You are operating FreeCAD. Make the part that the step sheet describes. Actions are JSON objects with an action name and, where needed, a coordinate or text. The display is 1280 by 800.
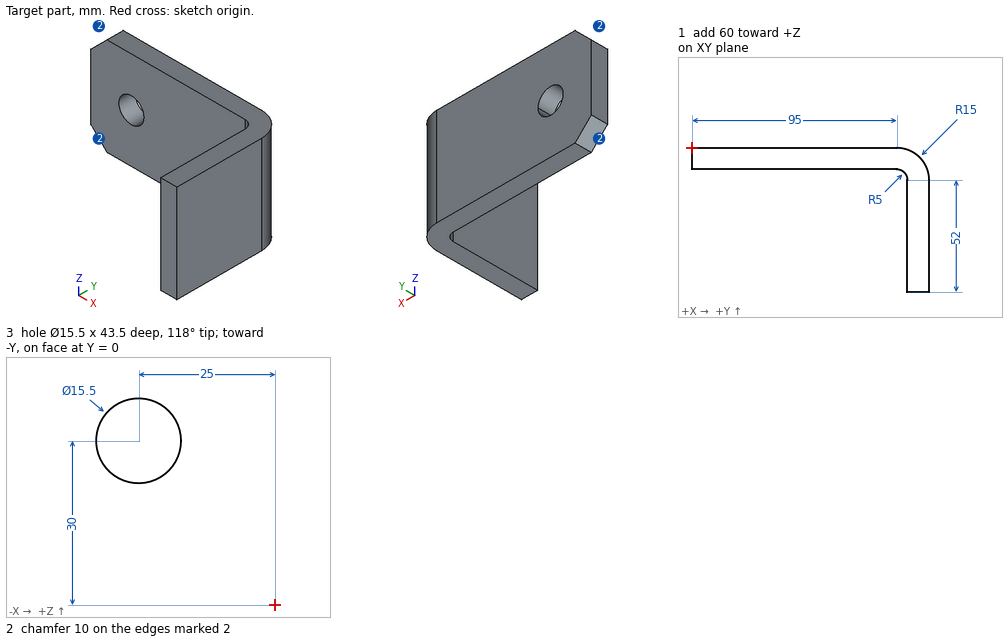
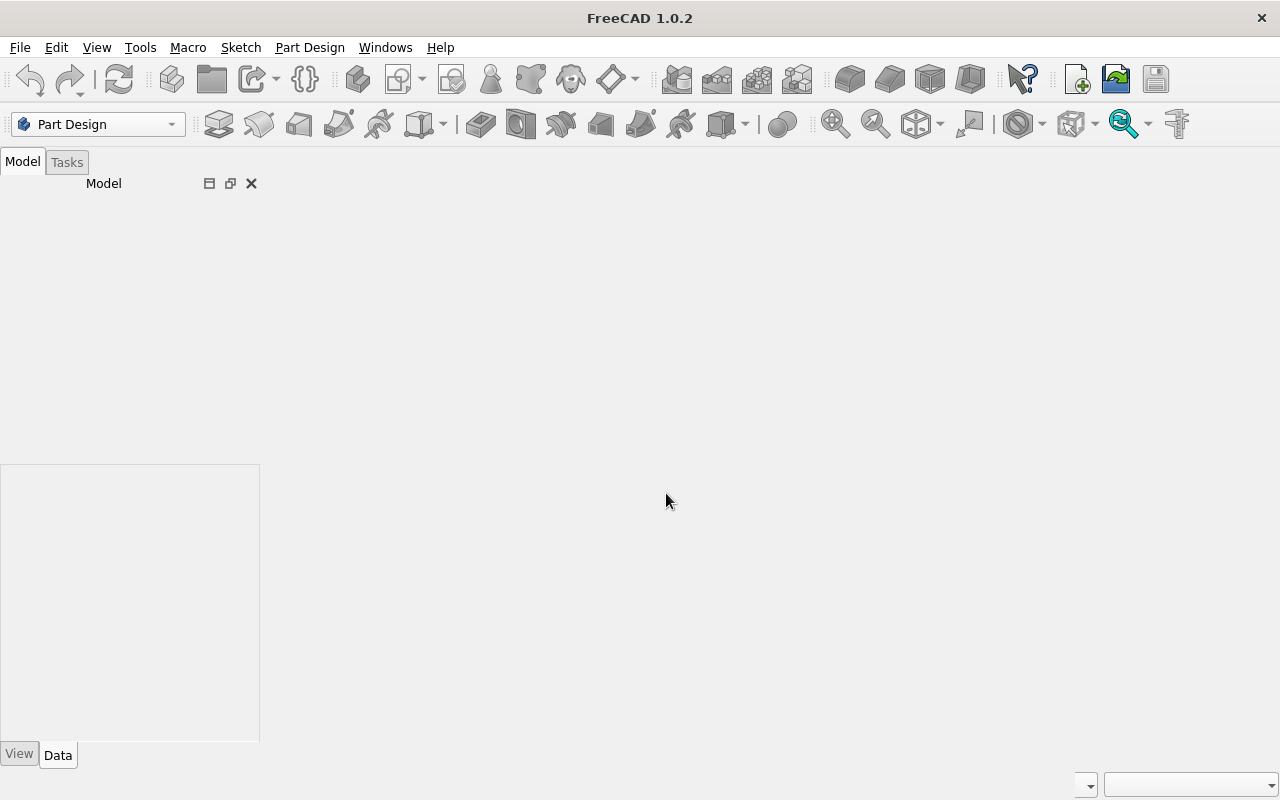
{"action": "left_click", "coordinate": [1076, 80]}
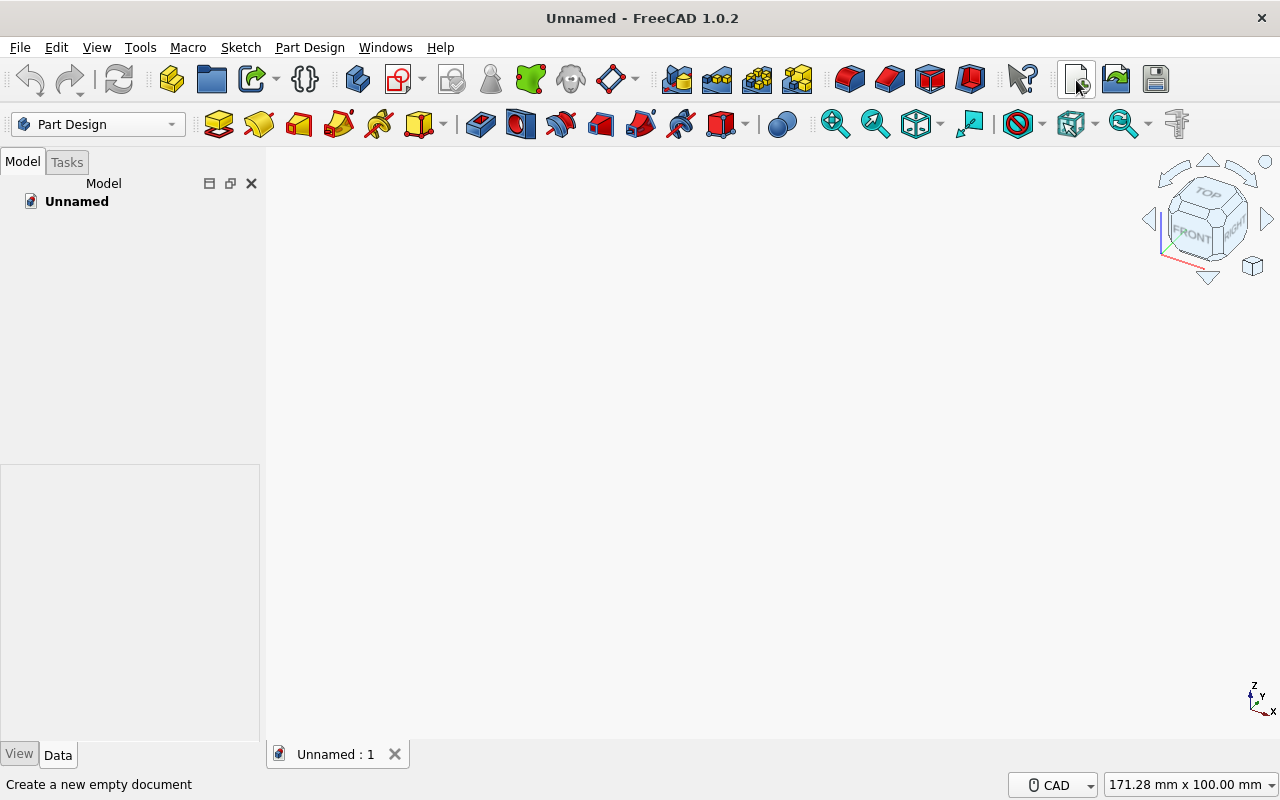
{"action": "left_click", "coordinate": [398, 80]}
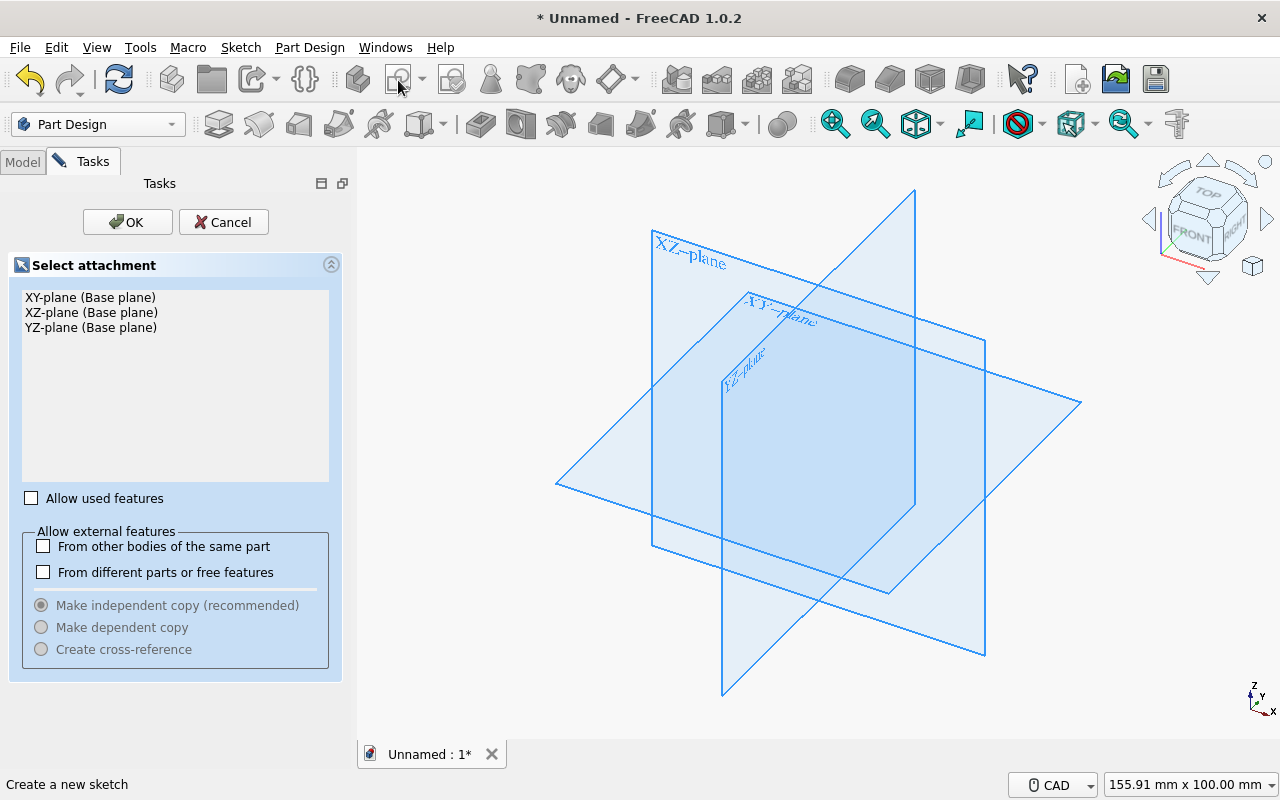
{"action": "left_click", "coordinate": [82, 298]}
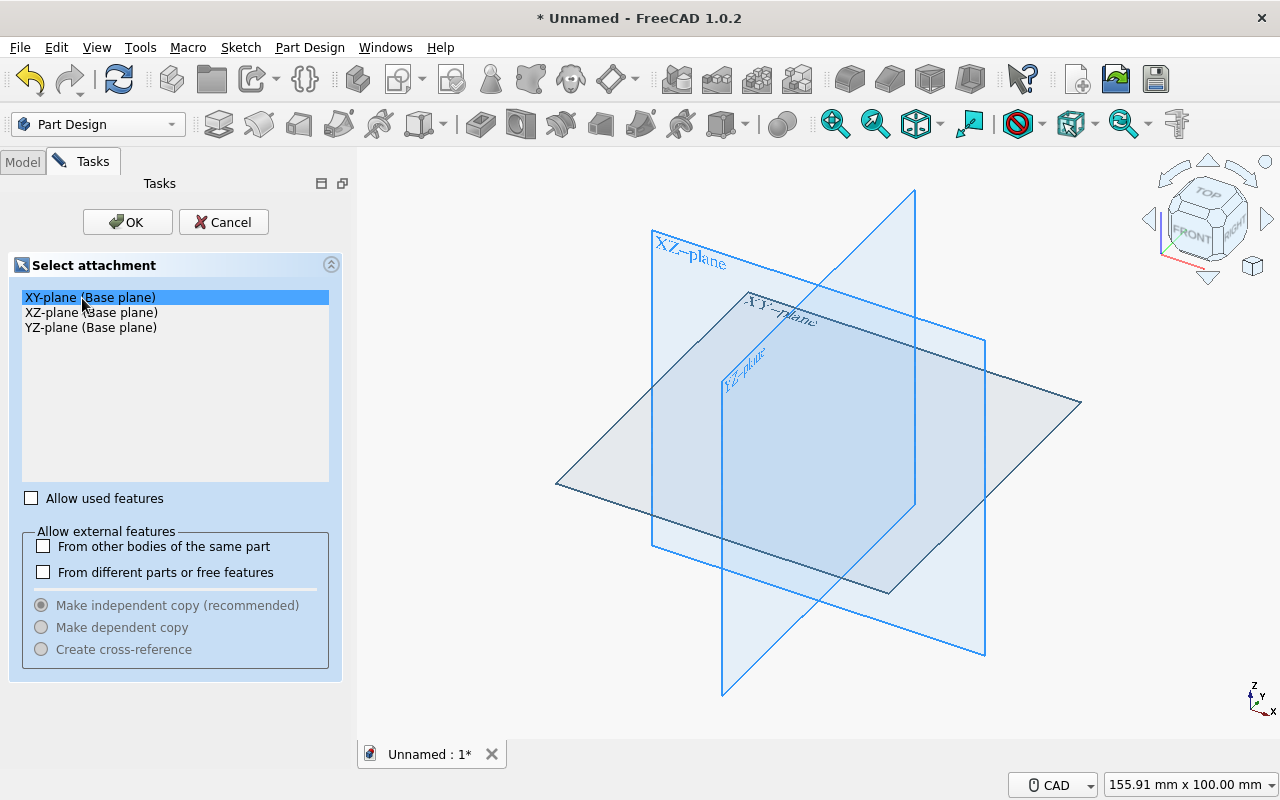
{"action": "left_click", "coordinate": [128, 222]}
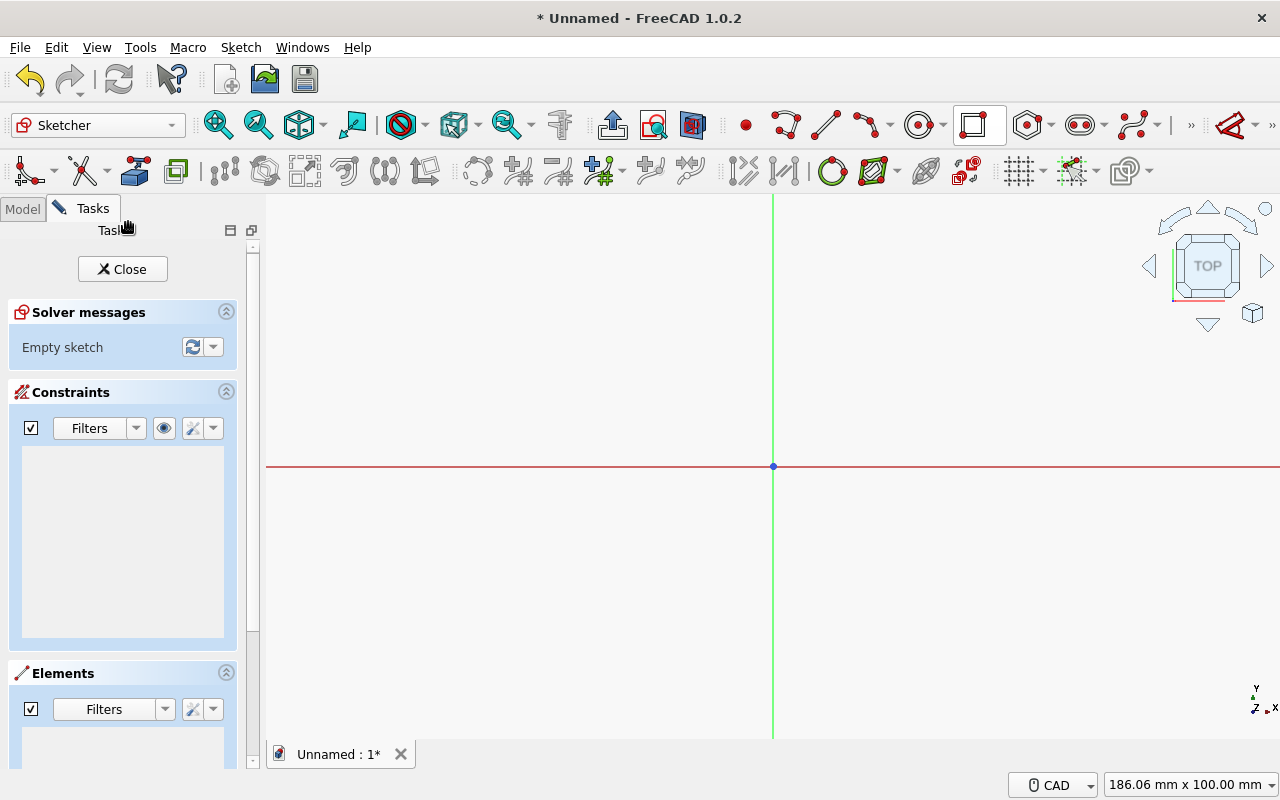
{"action": "scroll", "coordinate": [294, 222], "scroll_direction": "down", "scroll_amount": 2}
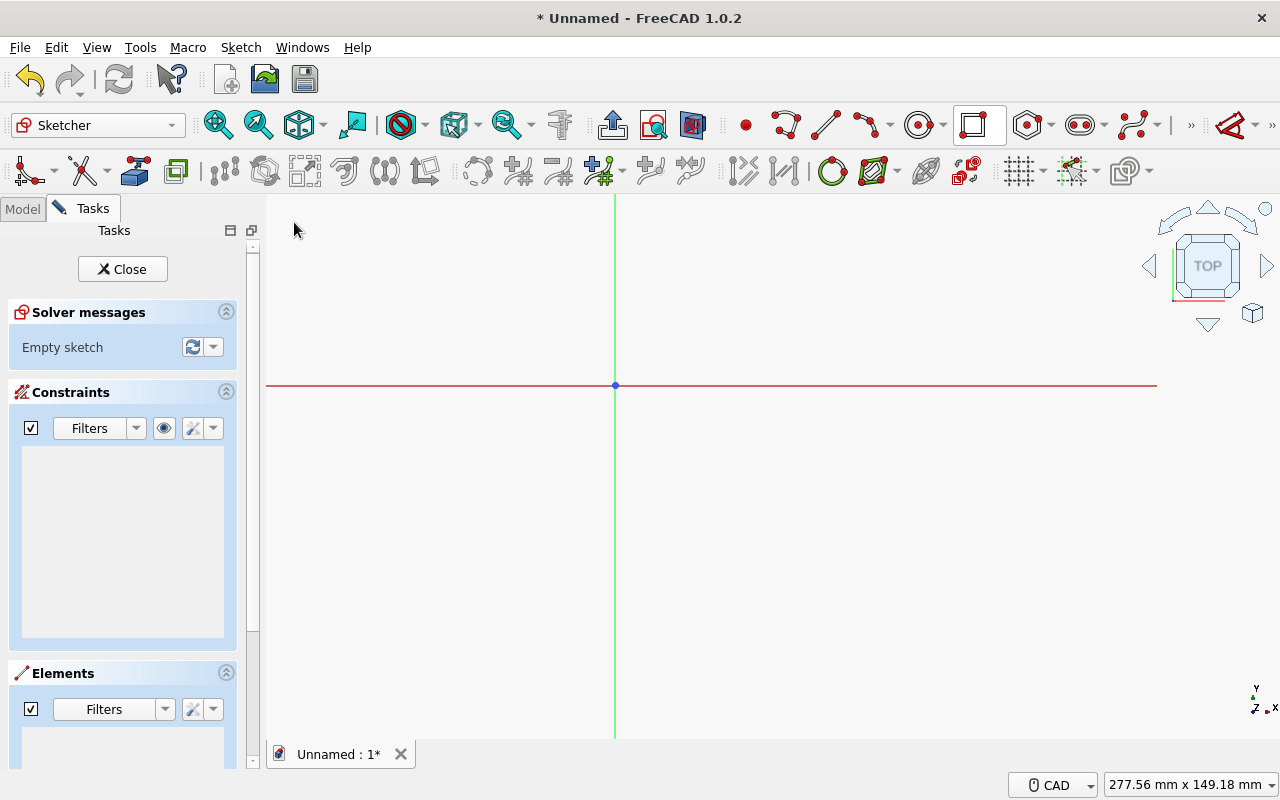
{"action": "scroll", "coordinate": [1043, 593], "scroll_direction": "up", "scroll_amount": 2}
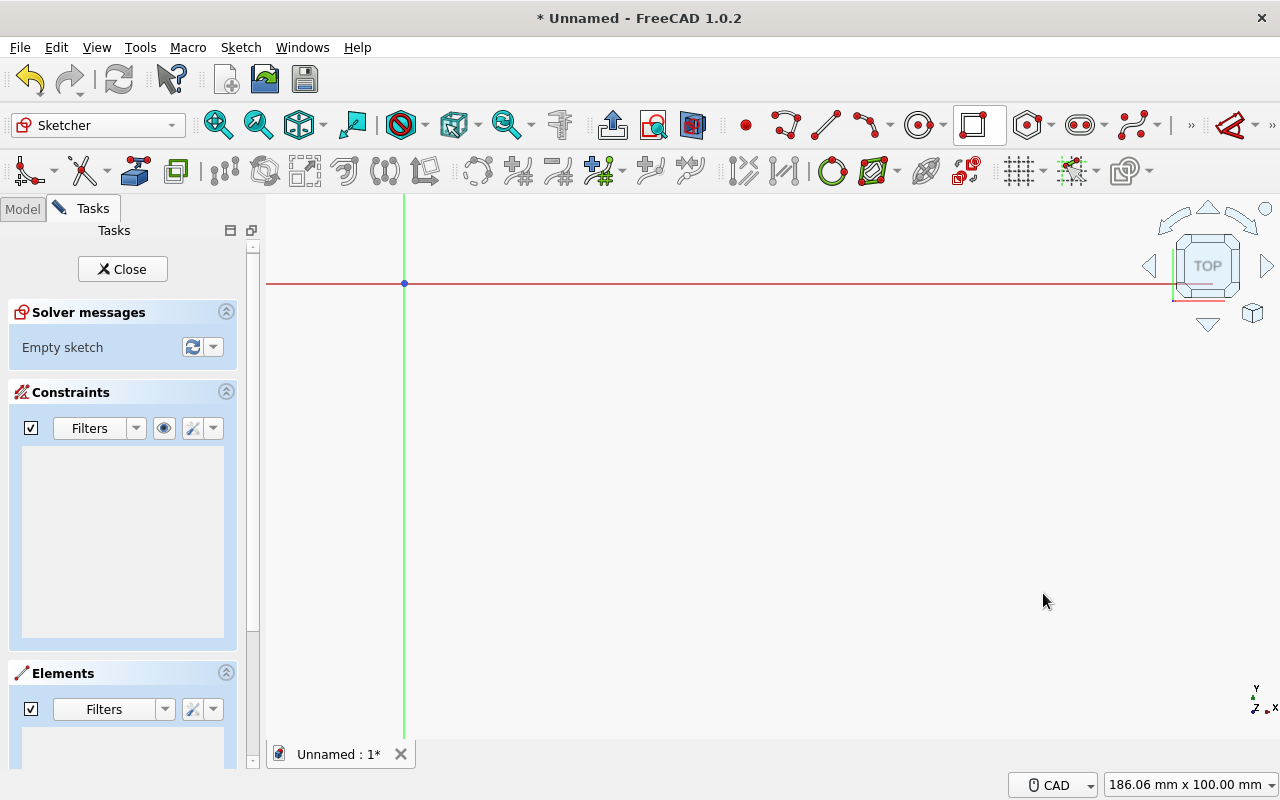
{"action": "left_click", "coordinate": [786, 126]}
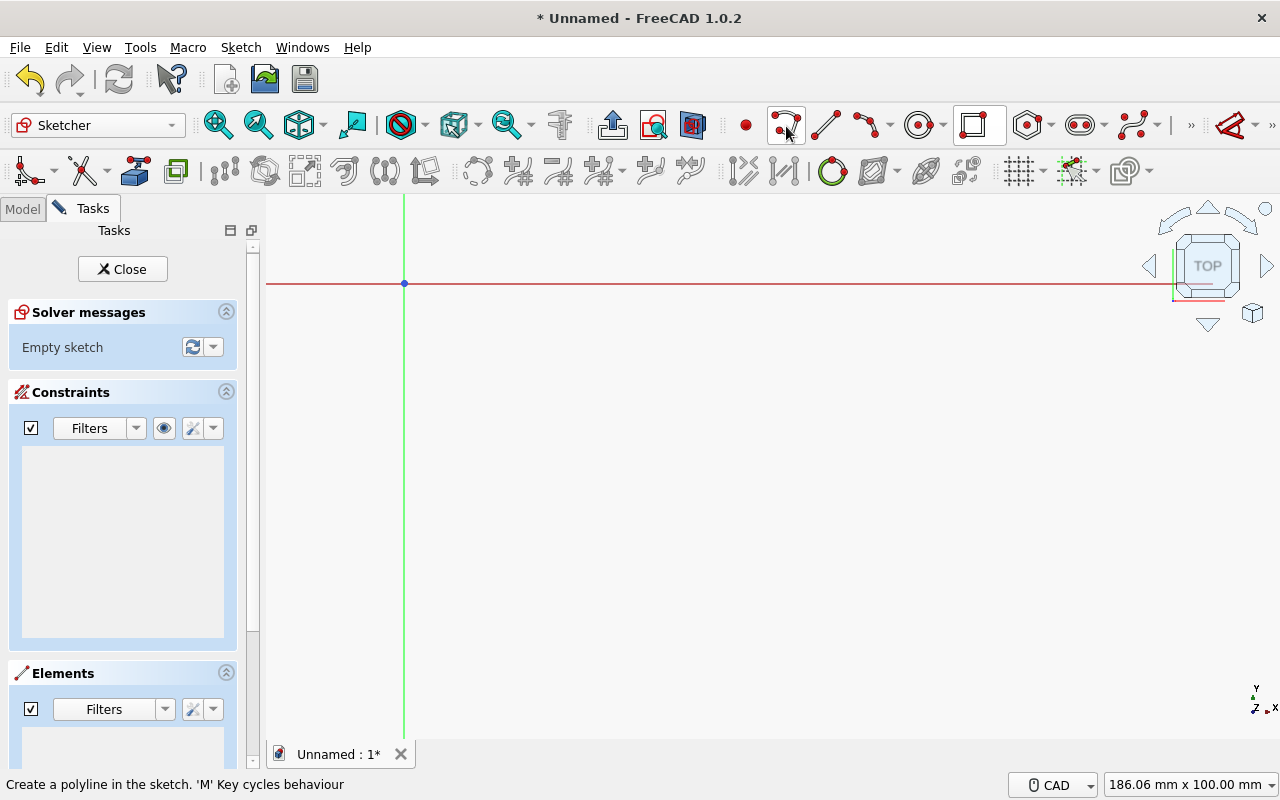
{"action": "left_click", "coordinate": [922, 284]}
{"action": "left_click", "coordinate": [404, 284]}
{"action": "left_click", "coordinate": [413, 338]}
{"action": "left_click", "coordinate": [922, 338]}
{"action": "right_click", "coordinate": [922, 338]}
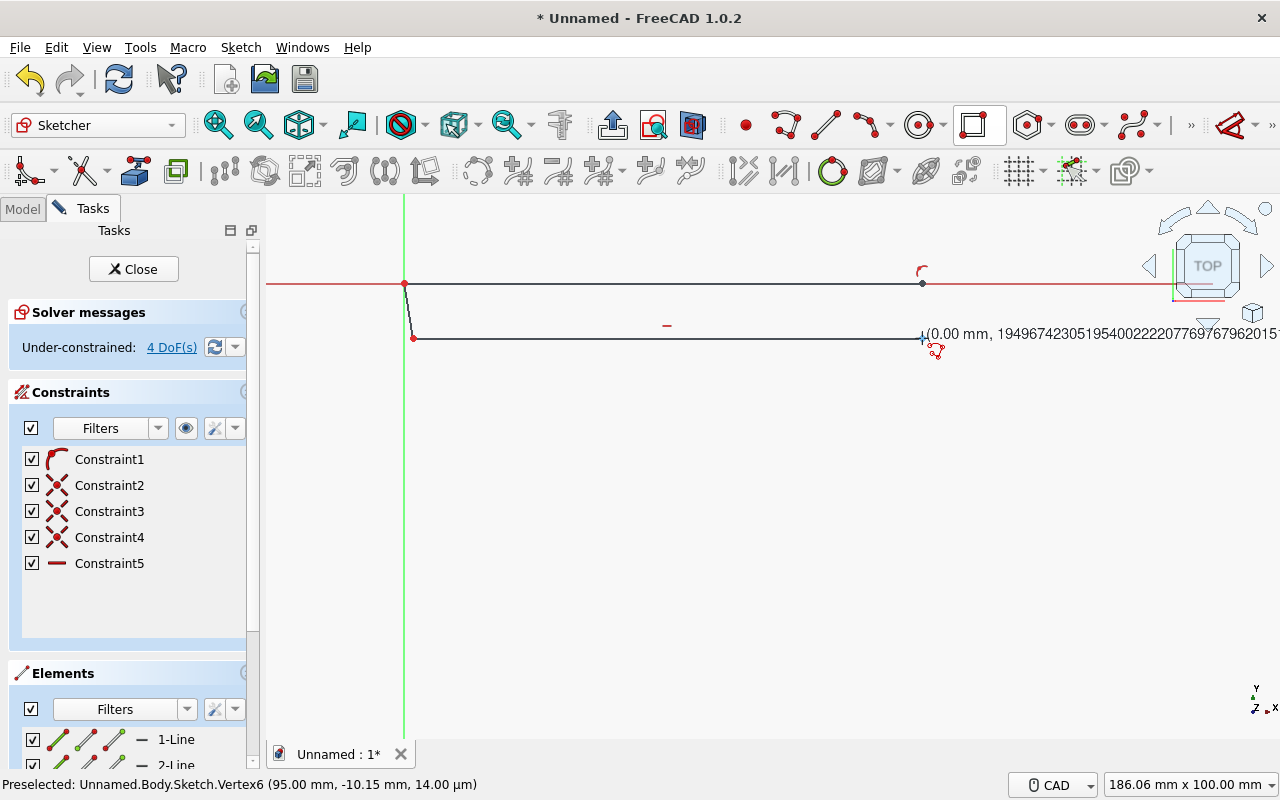
{"action": "left_click", "coordinate": [949, 365]}
{"action": "left_click", "coordinate": [949, 649]}
{"action": "left_click", "coordinate": [1004, 649]}
{"action": "left_click", "coordinate": [1004, 365]}
{"action": "right_click", "coordinate": [1004, 365]}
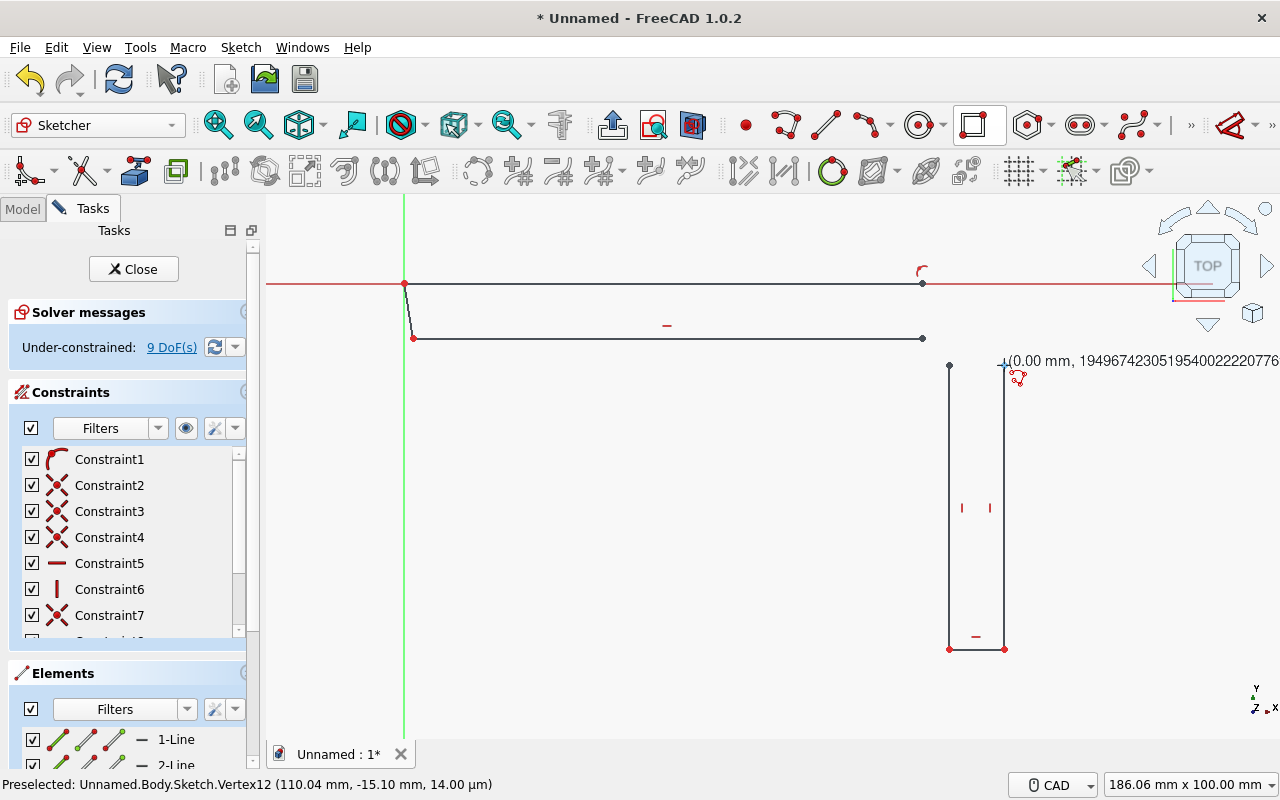
{"action": "left_click", "coordinate": [866, 126]}